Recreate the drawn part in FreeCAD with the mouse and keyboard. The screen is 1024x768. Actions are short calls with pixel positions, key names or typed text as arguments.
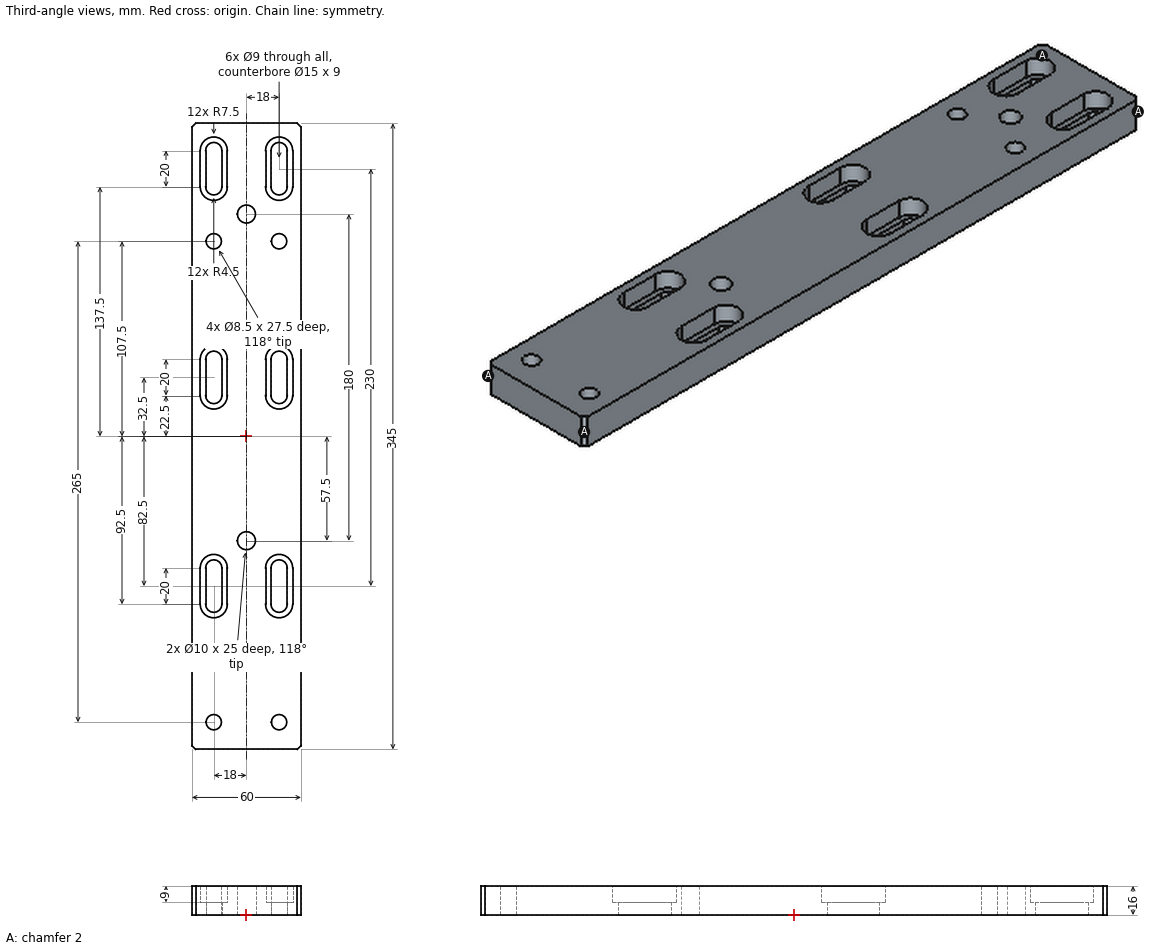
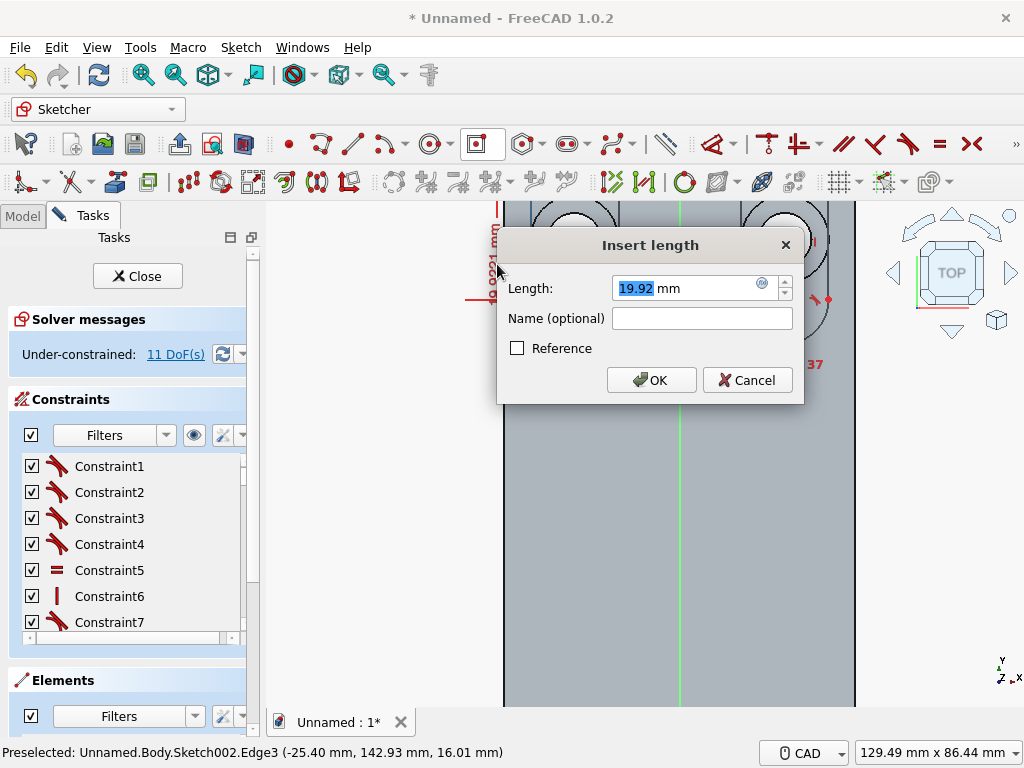
text(20)
key(Return)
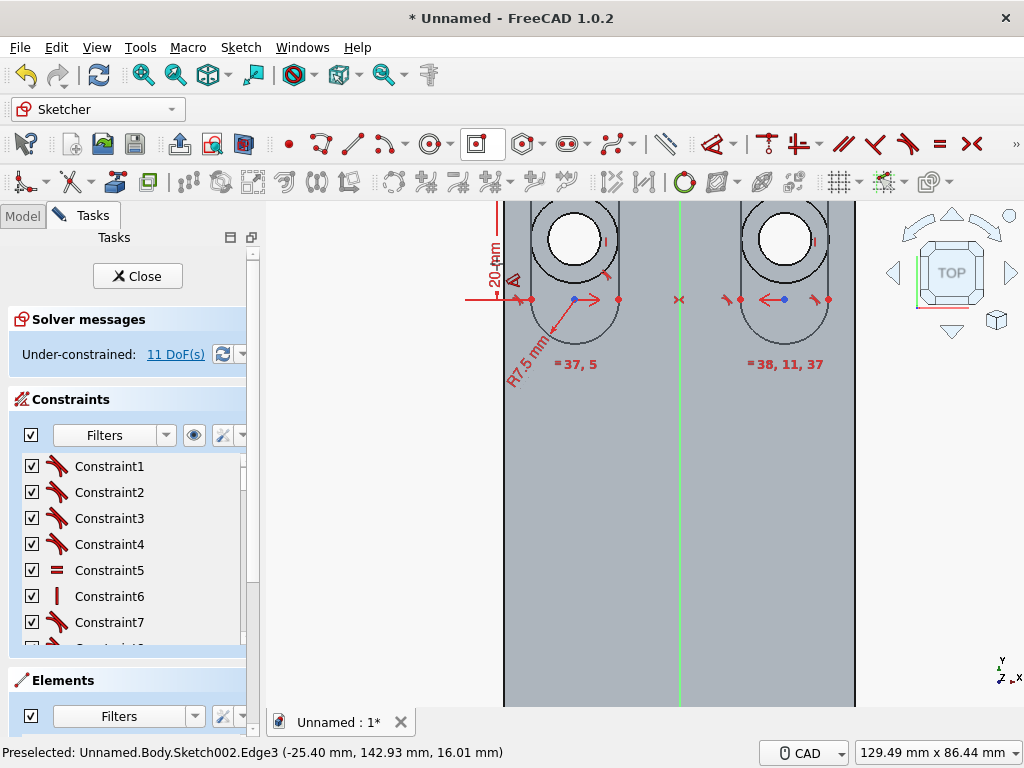
click(741, 265)
click(775, 264)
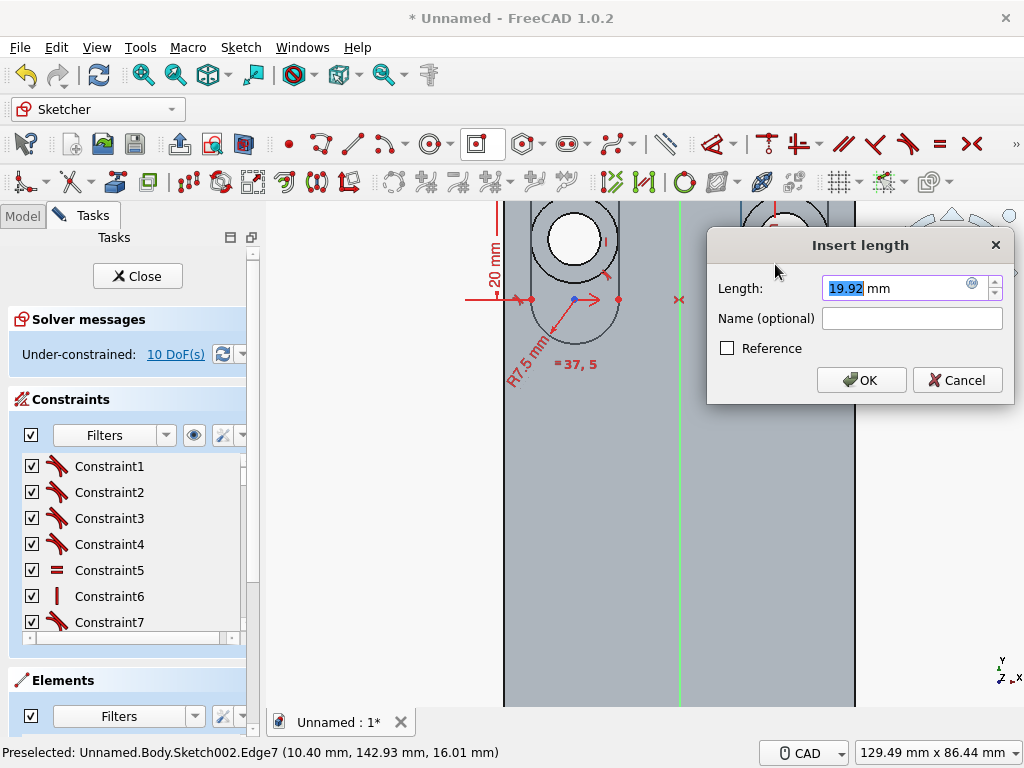
text(20)
key(Return)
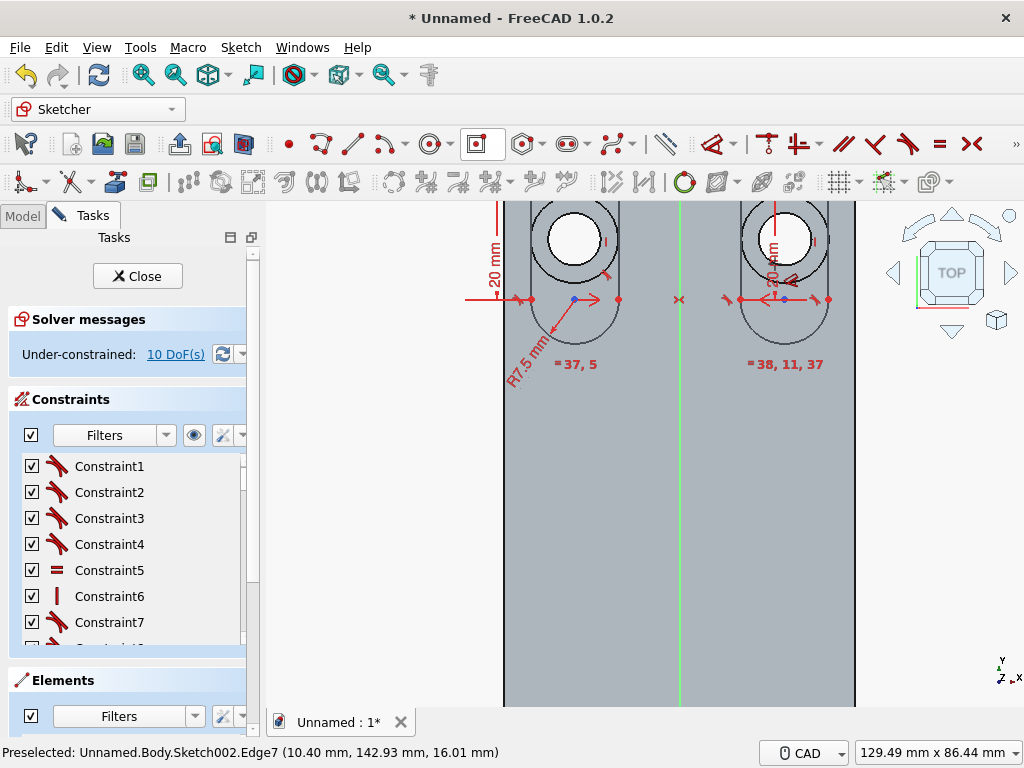
scroll(550, 338, down, 8)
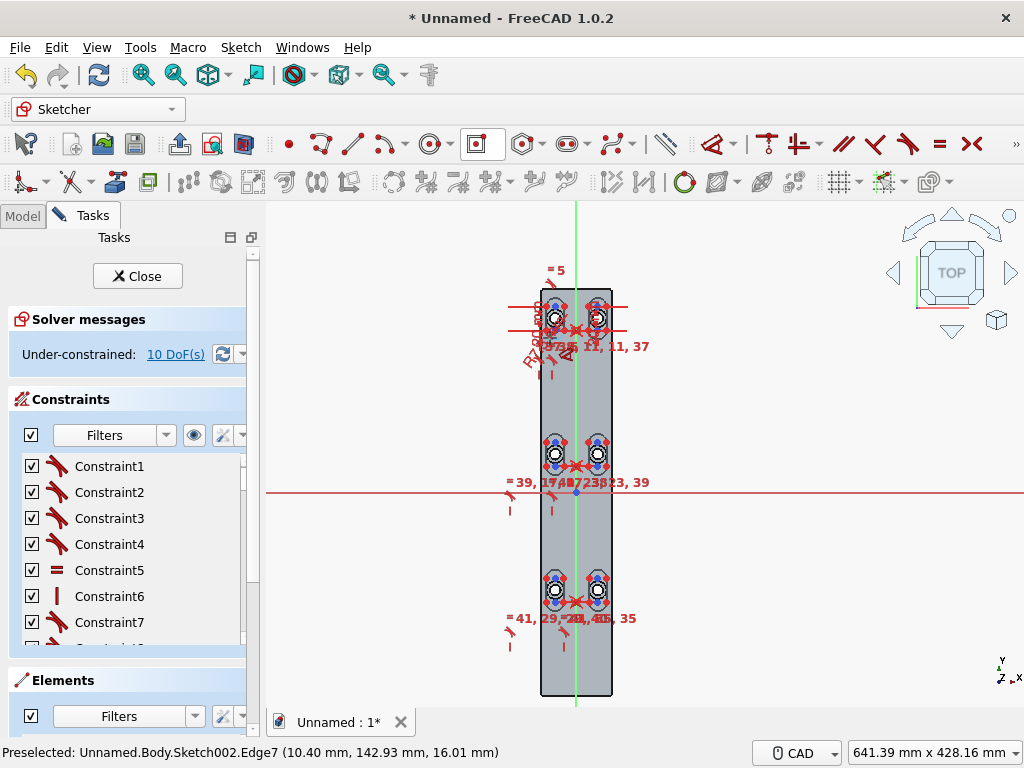
scroll(546, 459, up, 4)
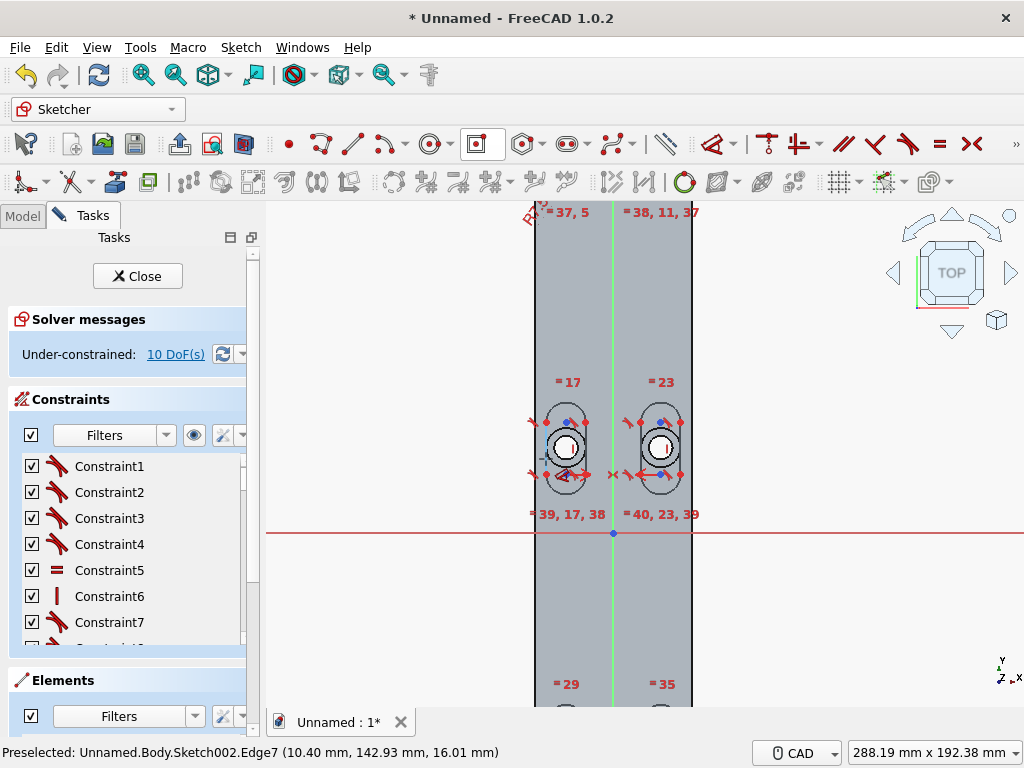
click(546, 459)
click(512, 448)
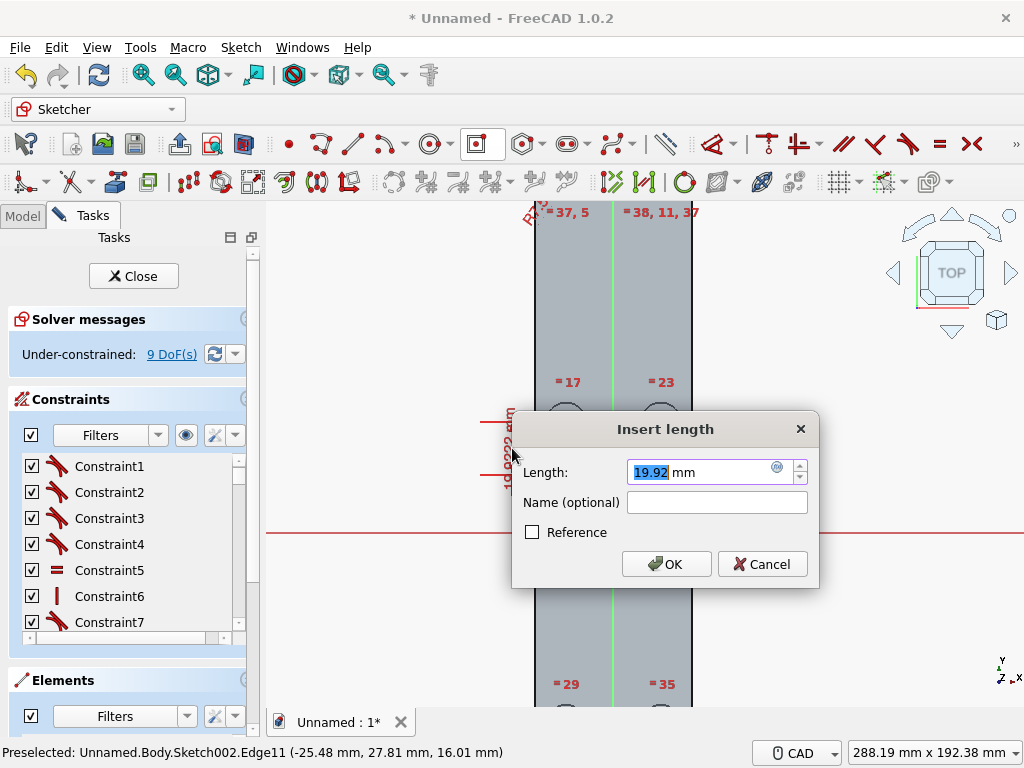
text(20)
key(Return)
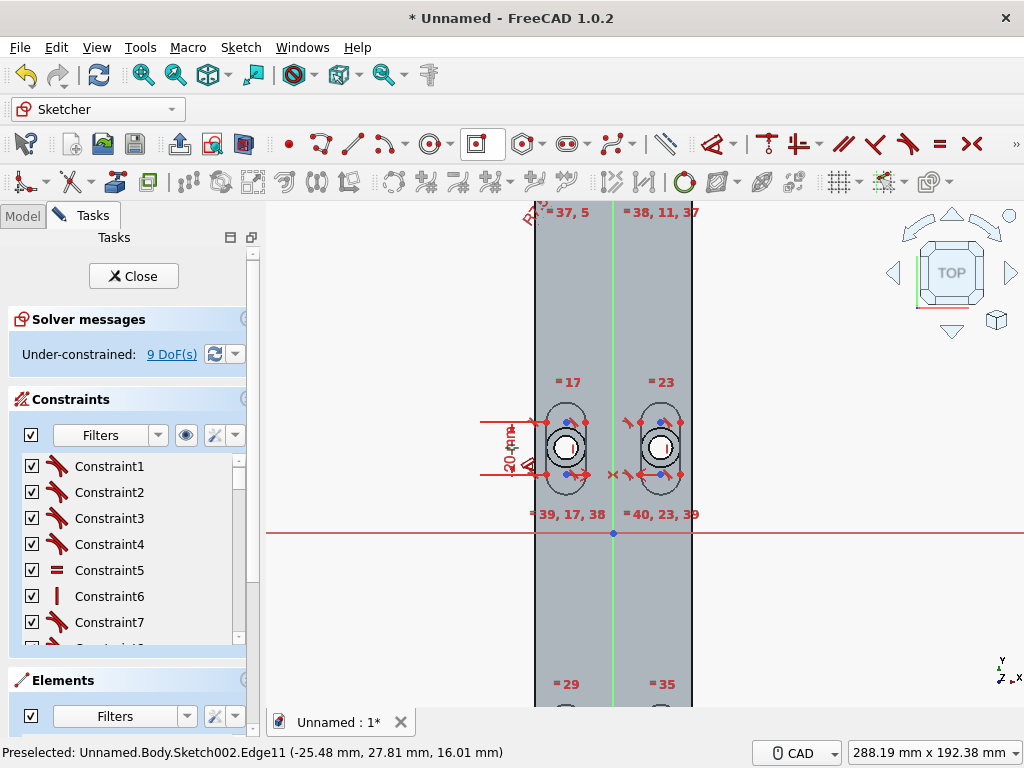
click(641, 459)
click(699, 449)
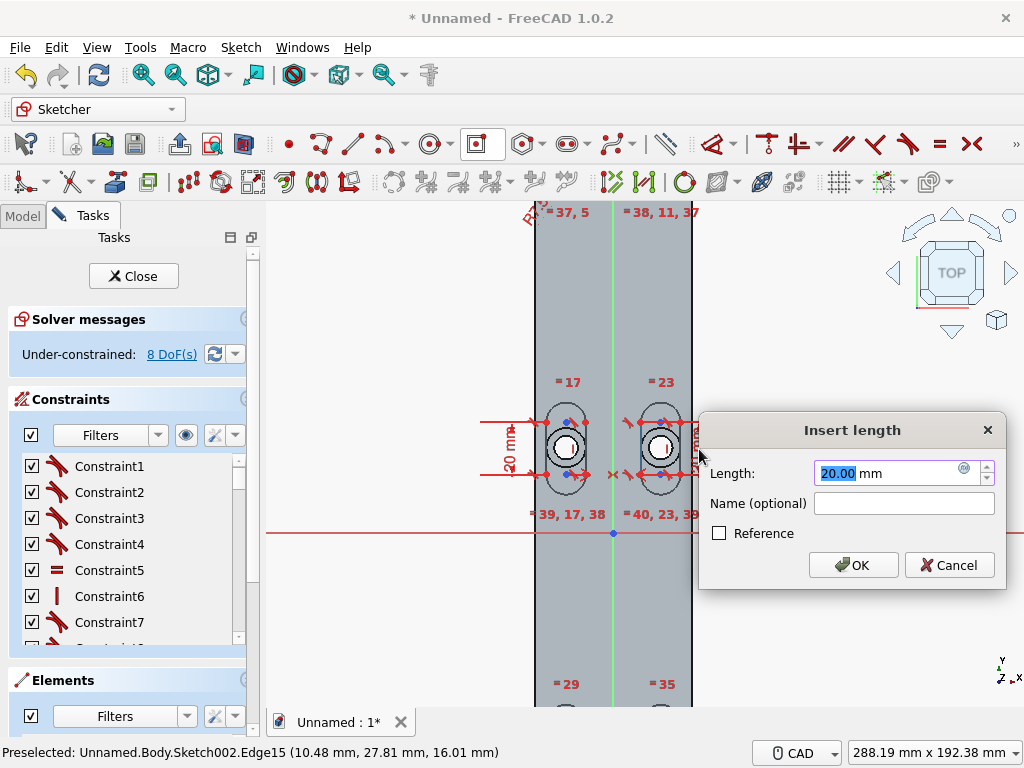
text(20)
key(Return)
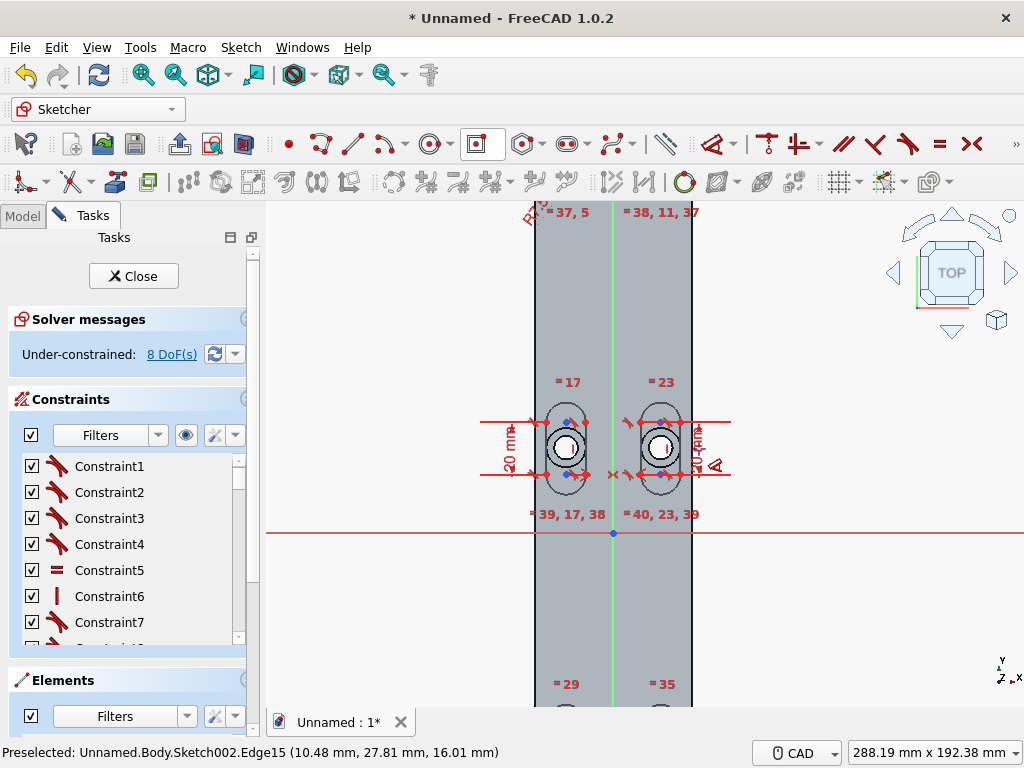
scroll(546, 459, down, 4)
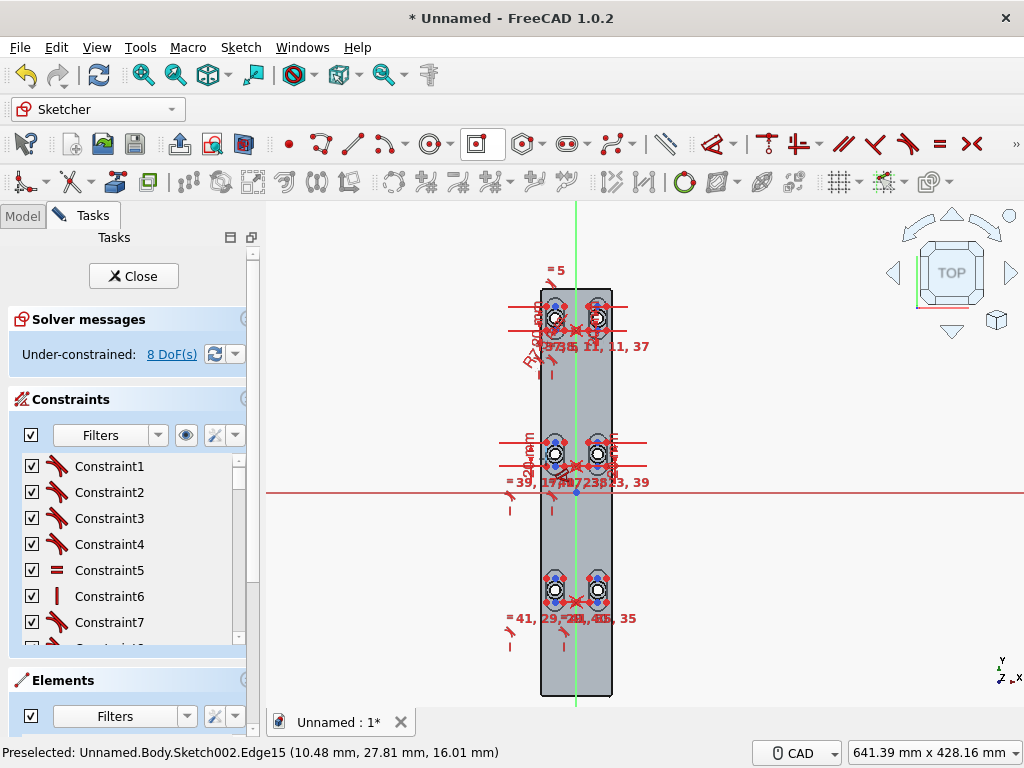
scroll(546, 595, up, 4)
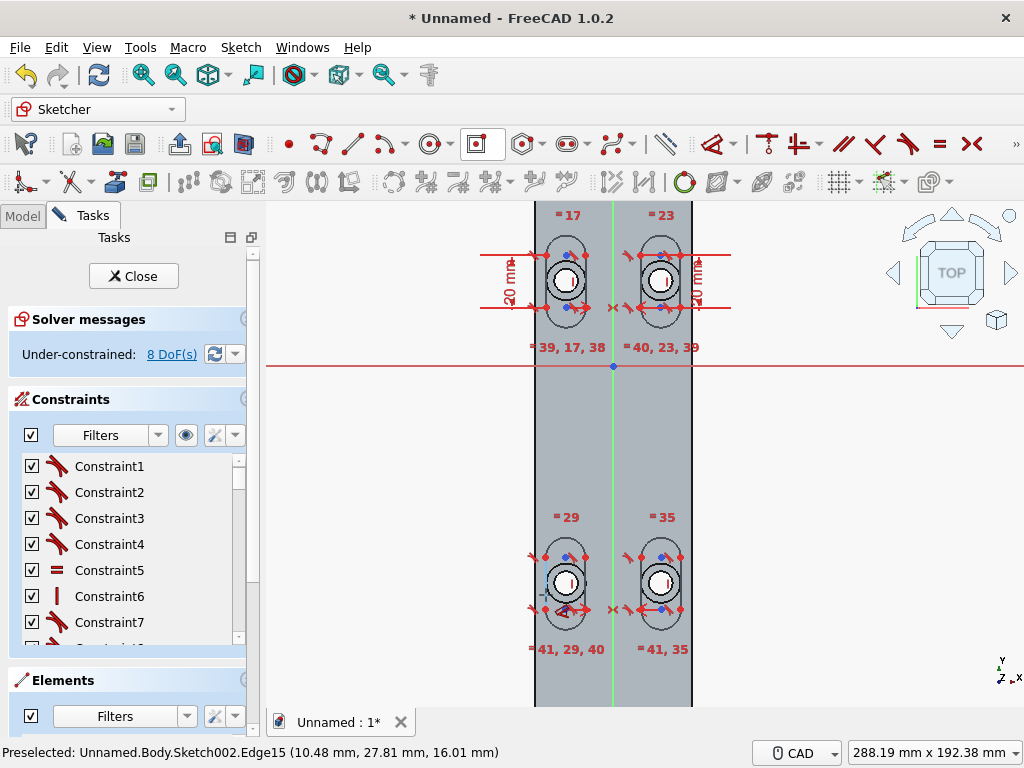
click(546, 594)
click(512, 584)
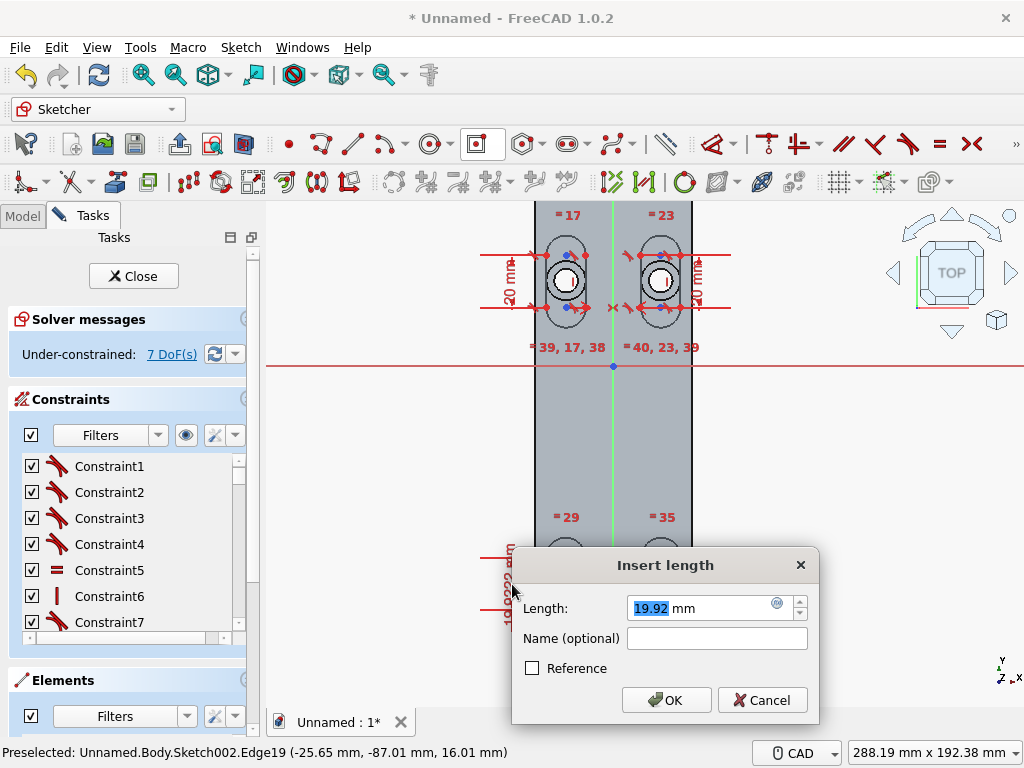
text(20)
key(Return)